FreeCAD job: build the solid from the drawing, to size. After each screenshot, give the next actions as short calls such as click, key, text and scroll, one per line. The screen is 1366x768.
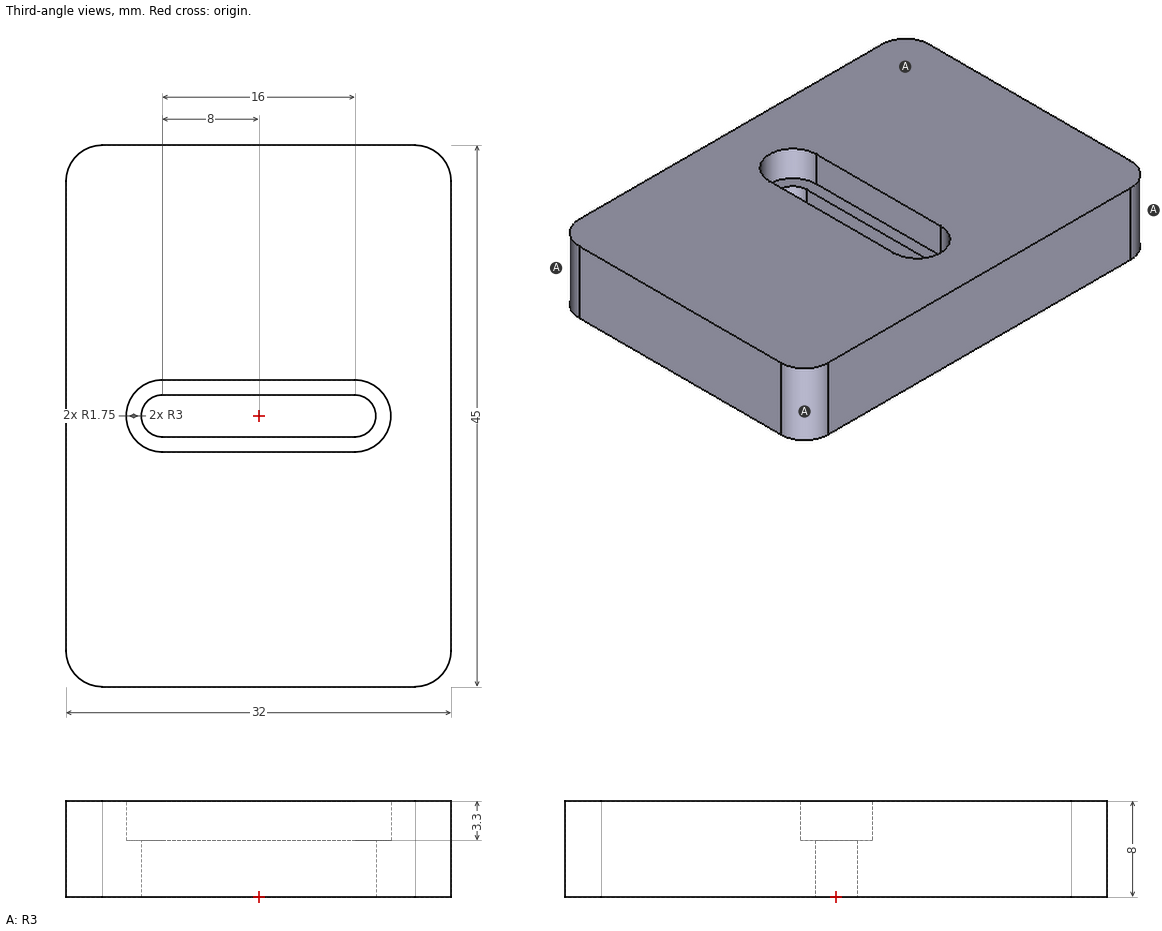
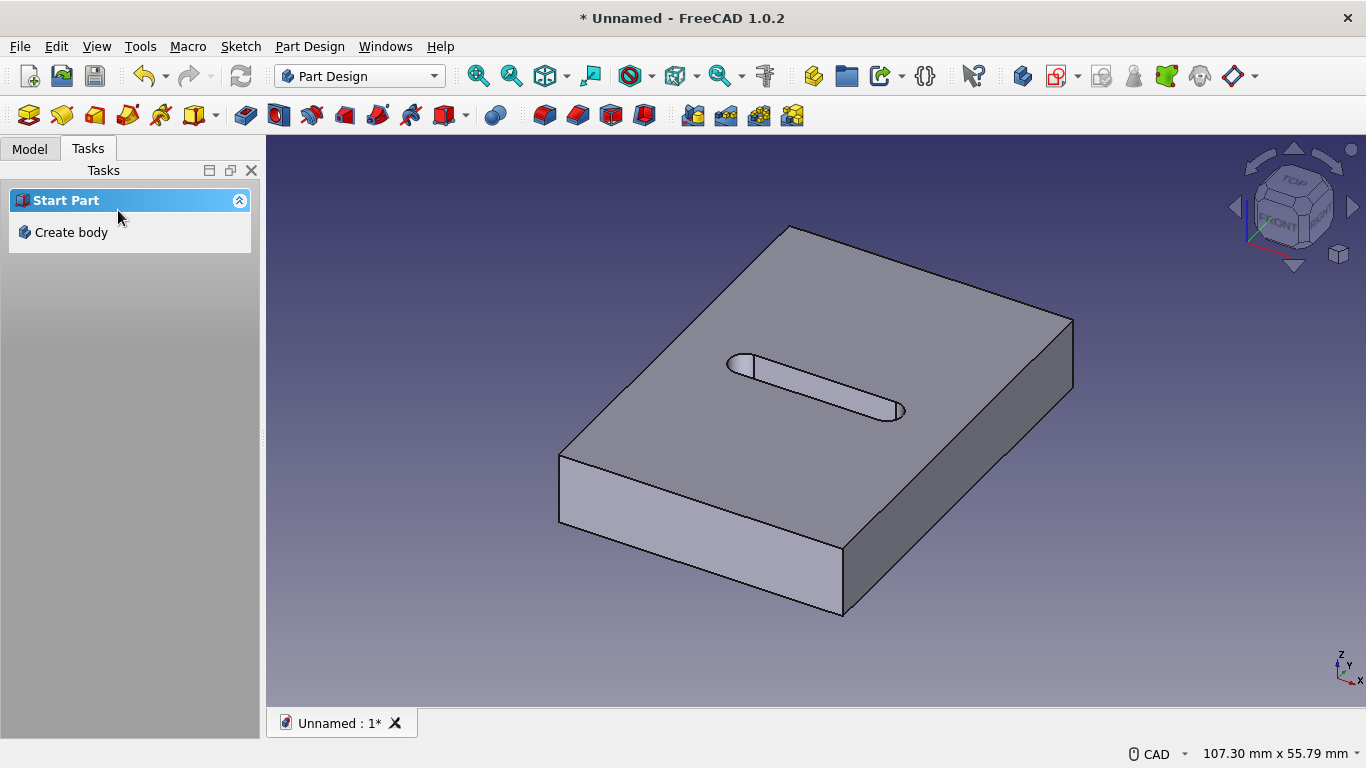
click(922, 334)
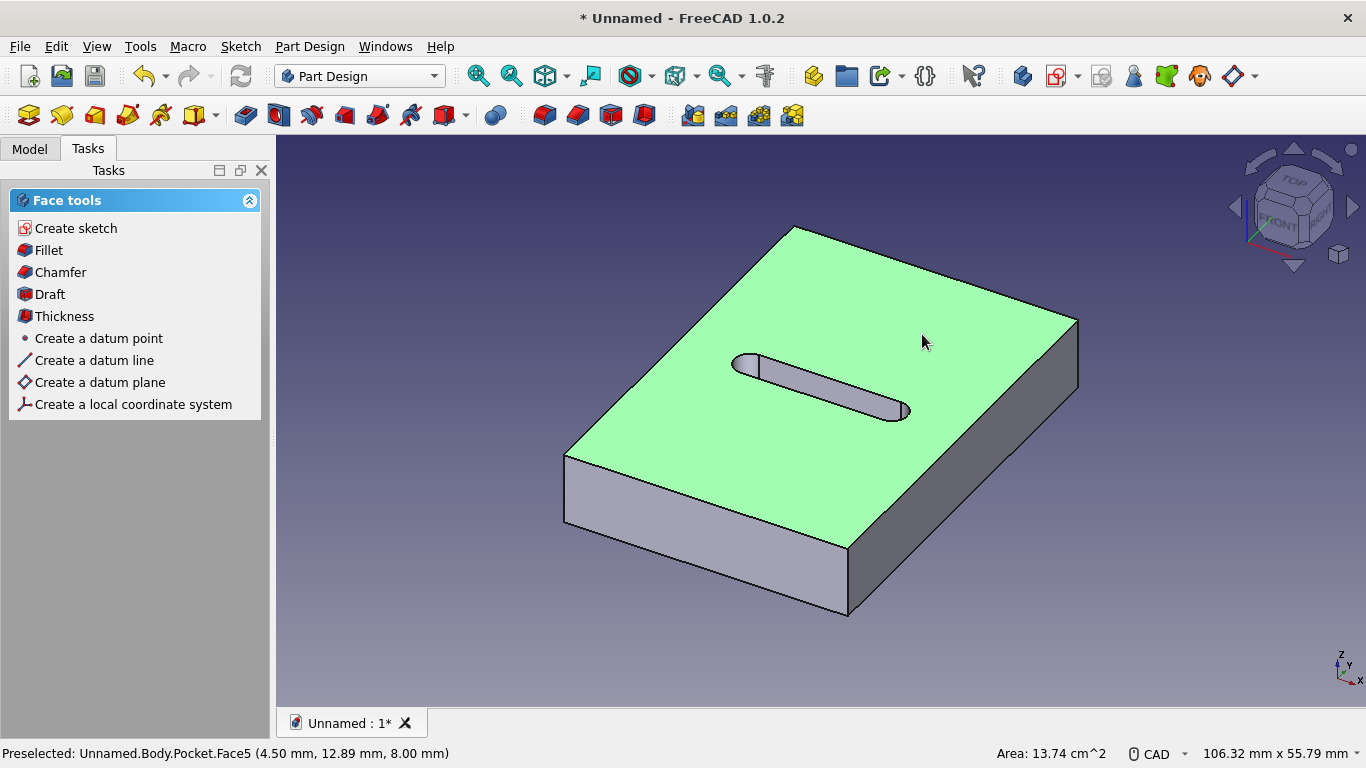
click(1056, 76)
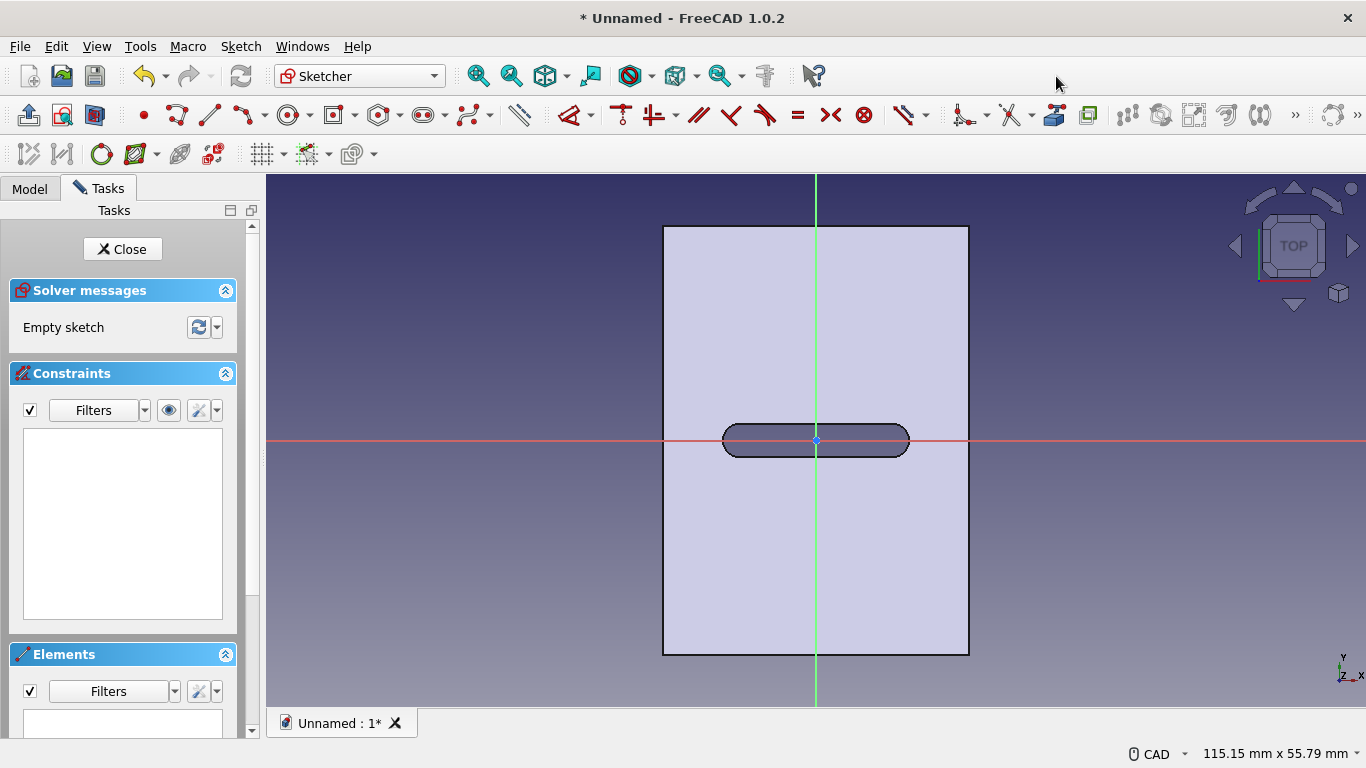
scroll(846, 440, up, 6)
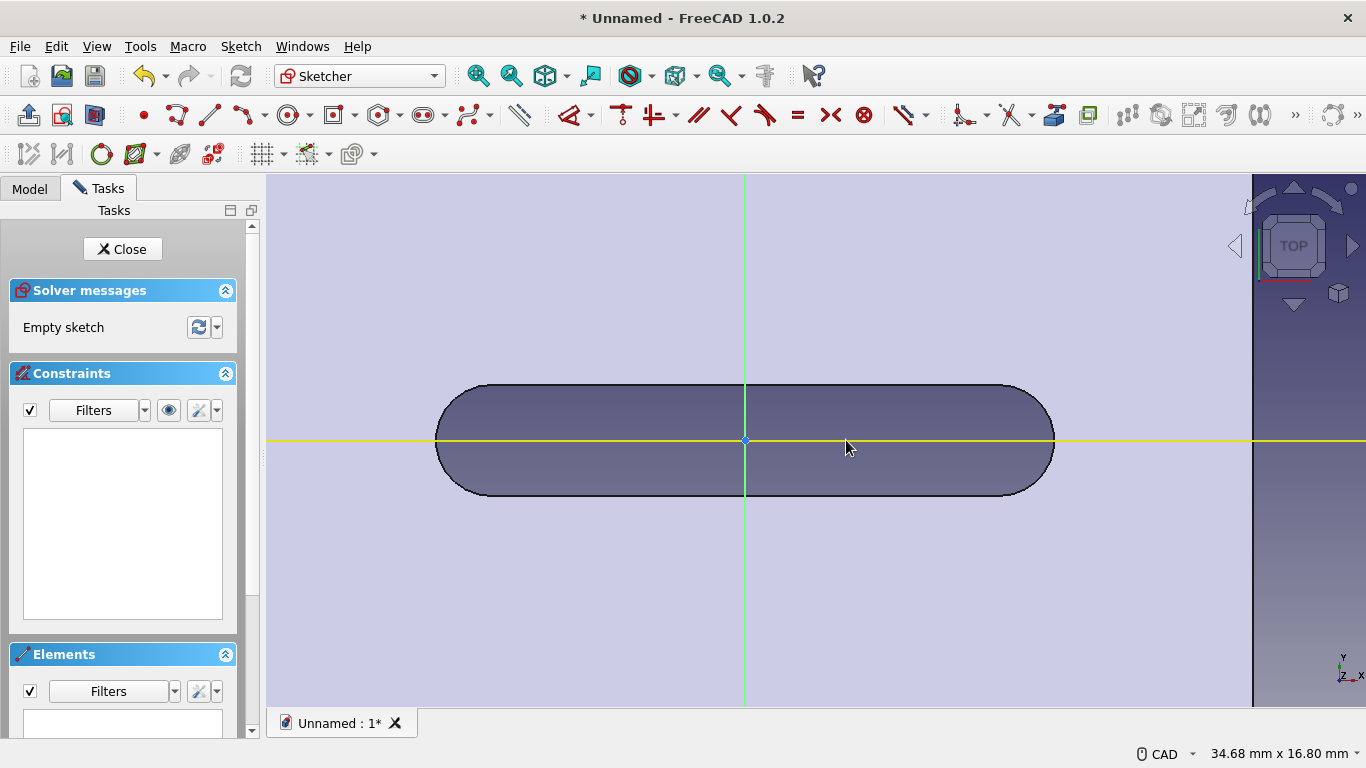
click(422, 116)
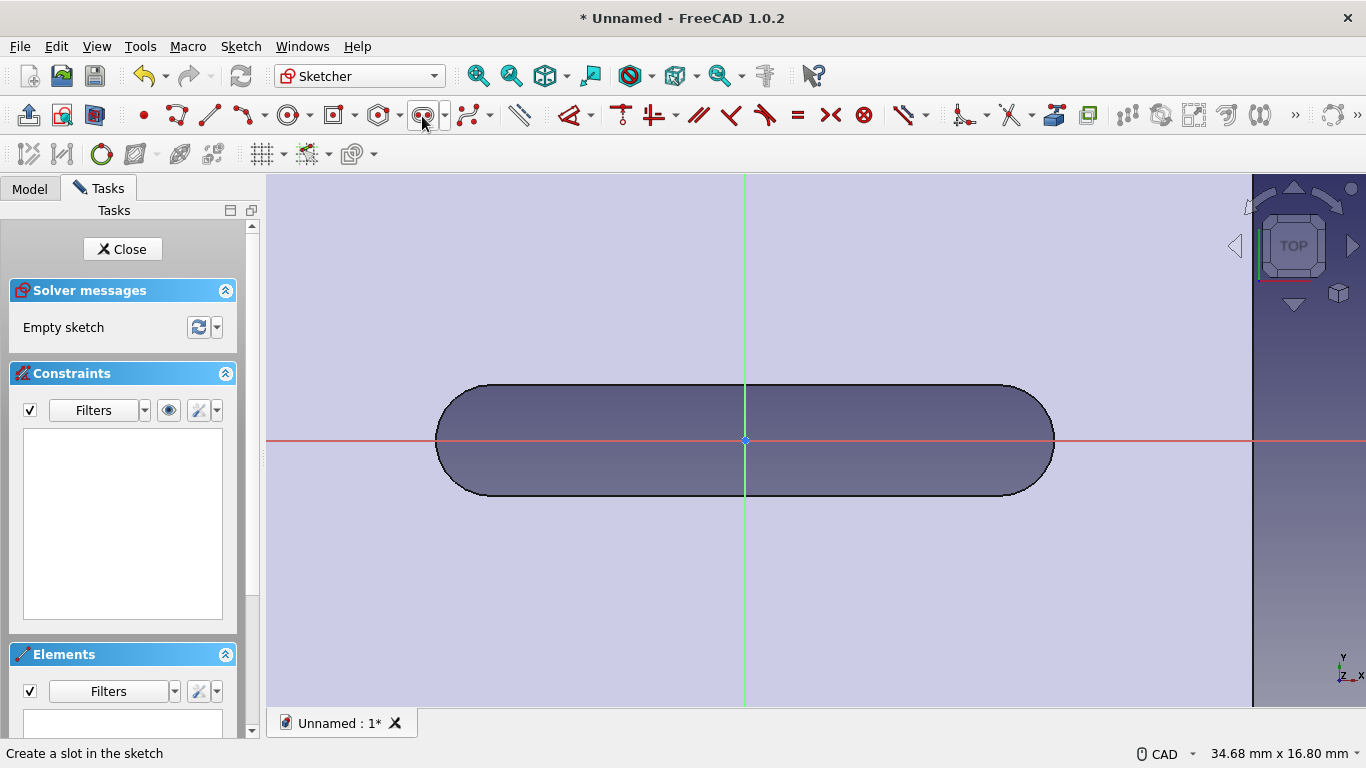
click(491, 440)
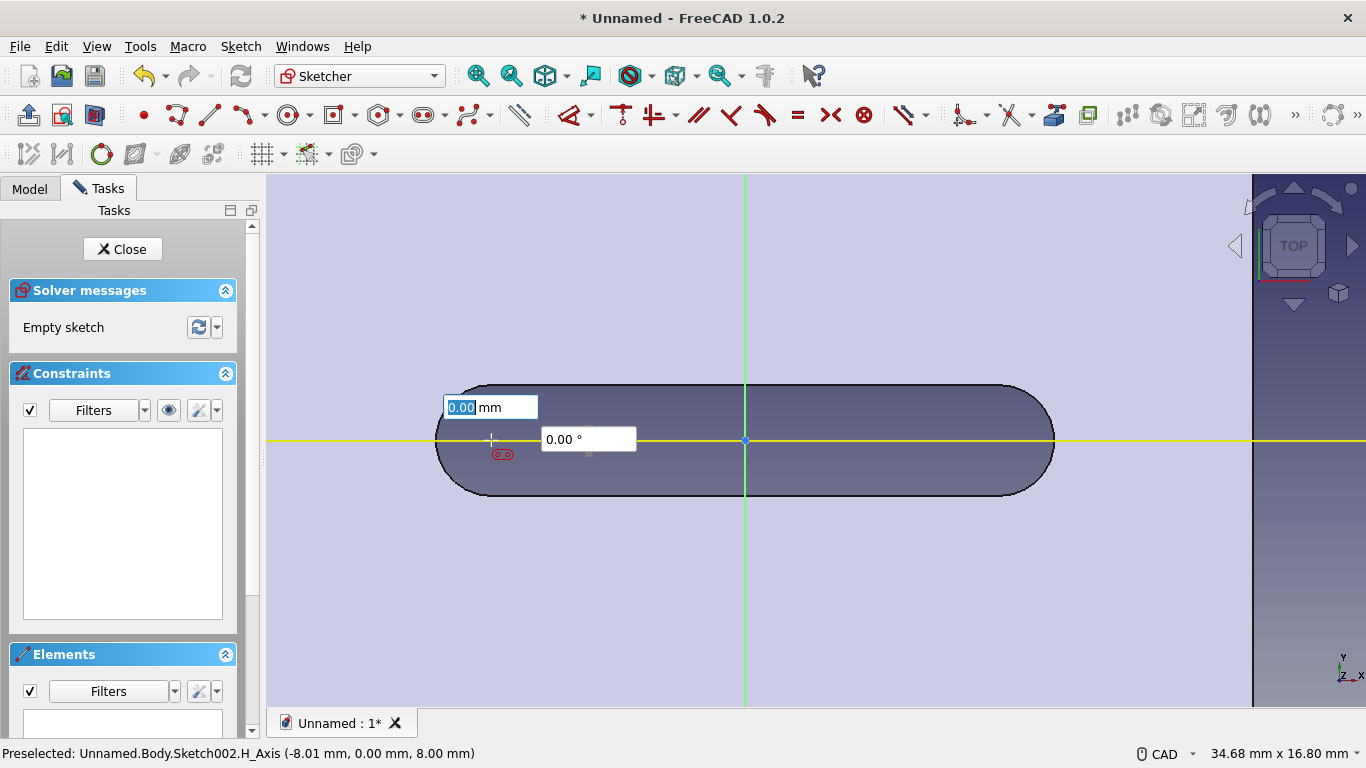
click(999, 432)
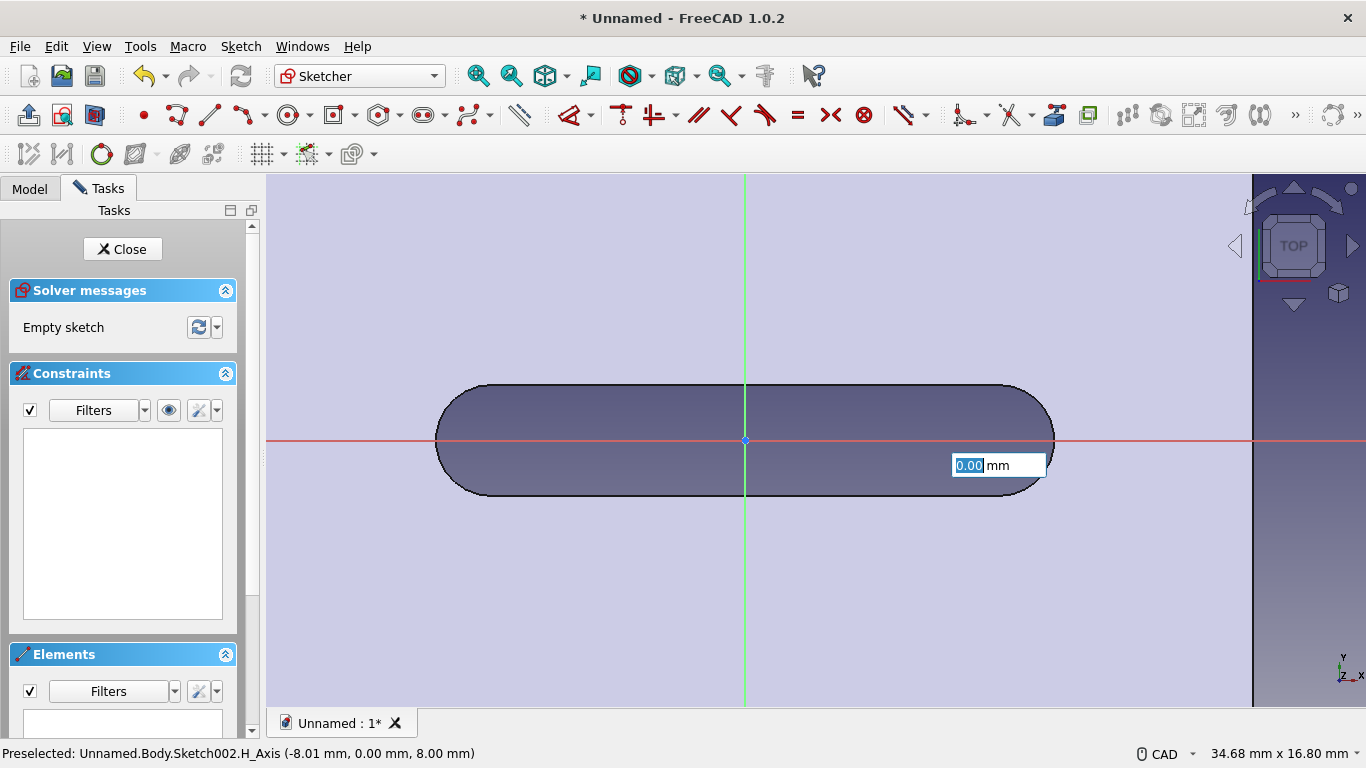
click(821, 345)
key(Escape)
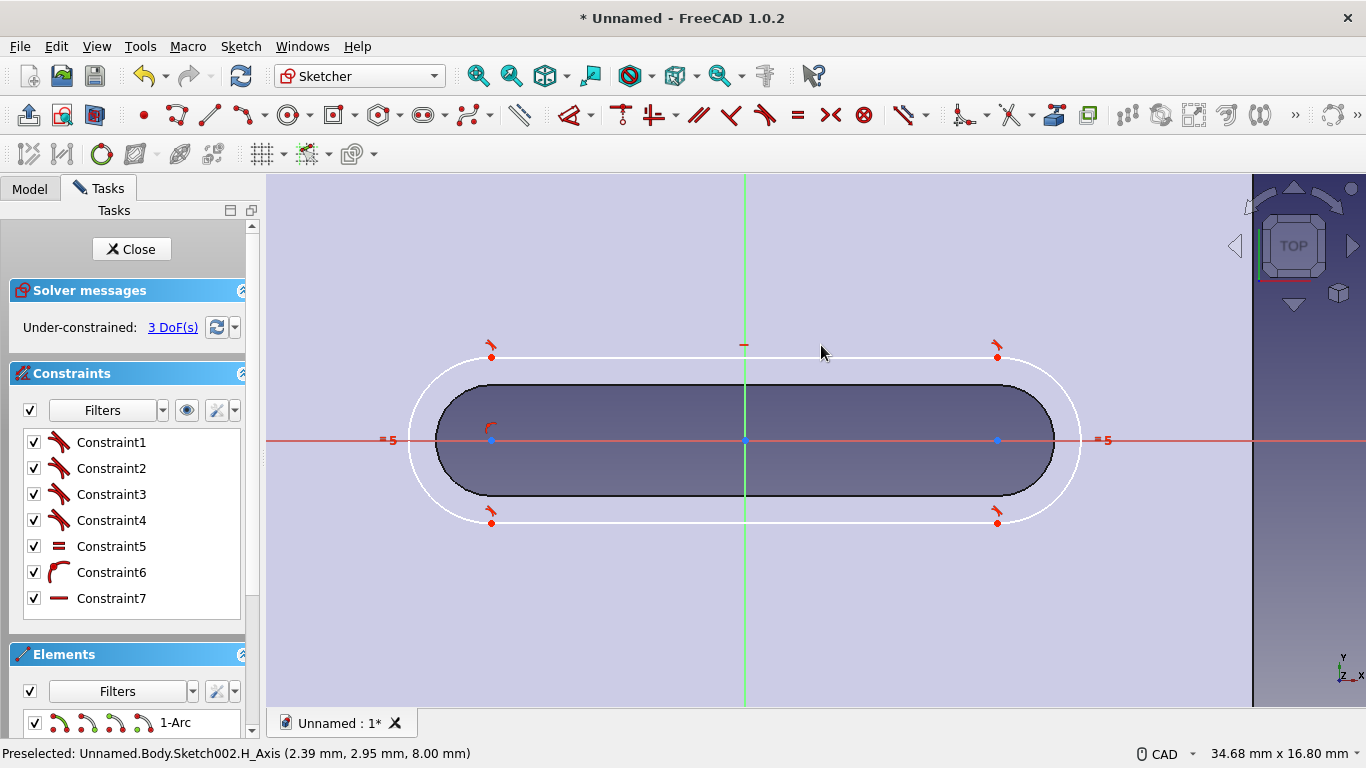
click(568, 116)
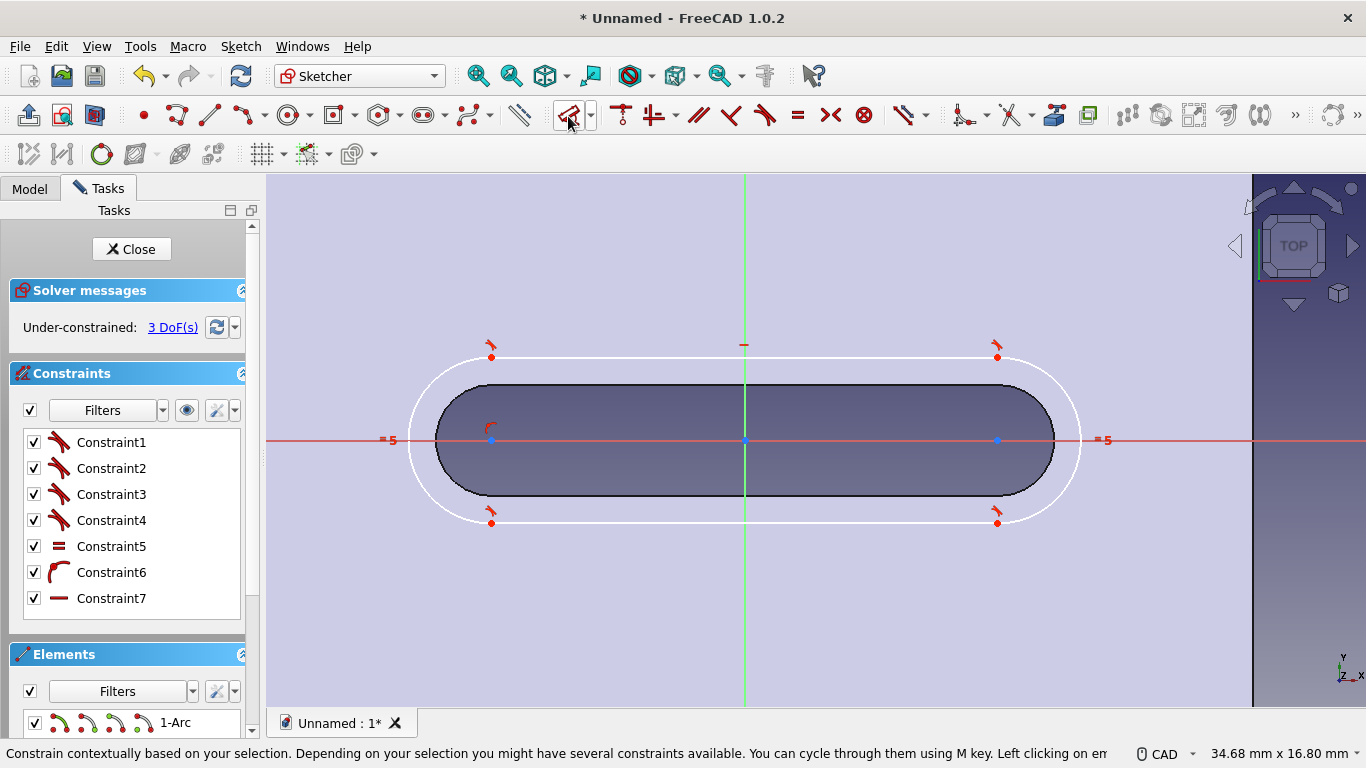
click(424, 392)
click(398, 373)